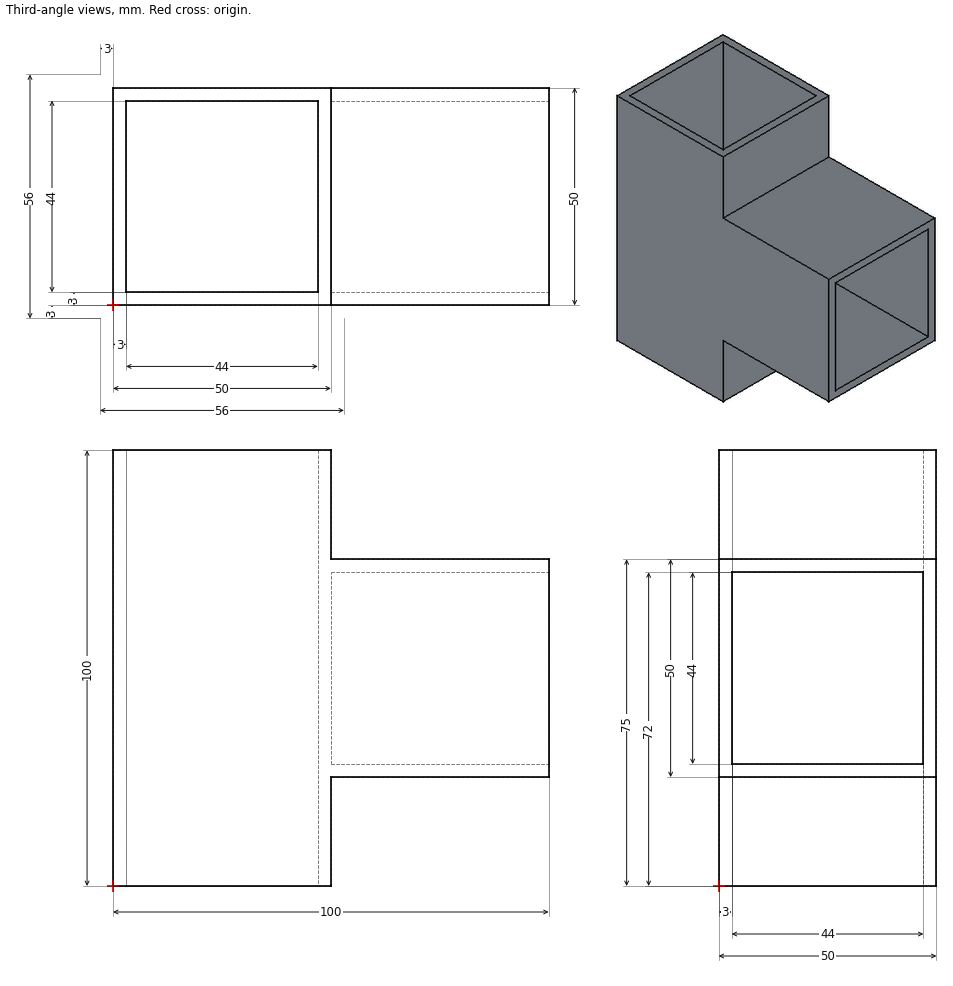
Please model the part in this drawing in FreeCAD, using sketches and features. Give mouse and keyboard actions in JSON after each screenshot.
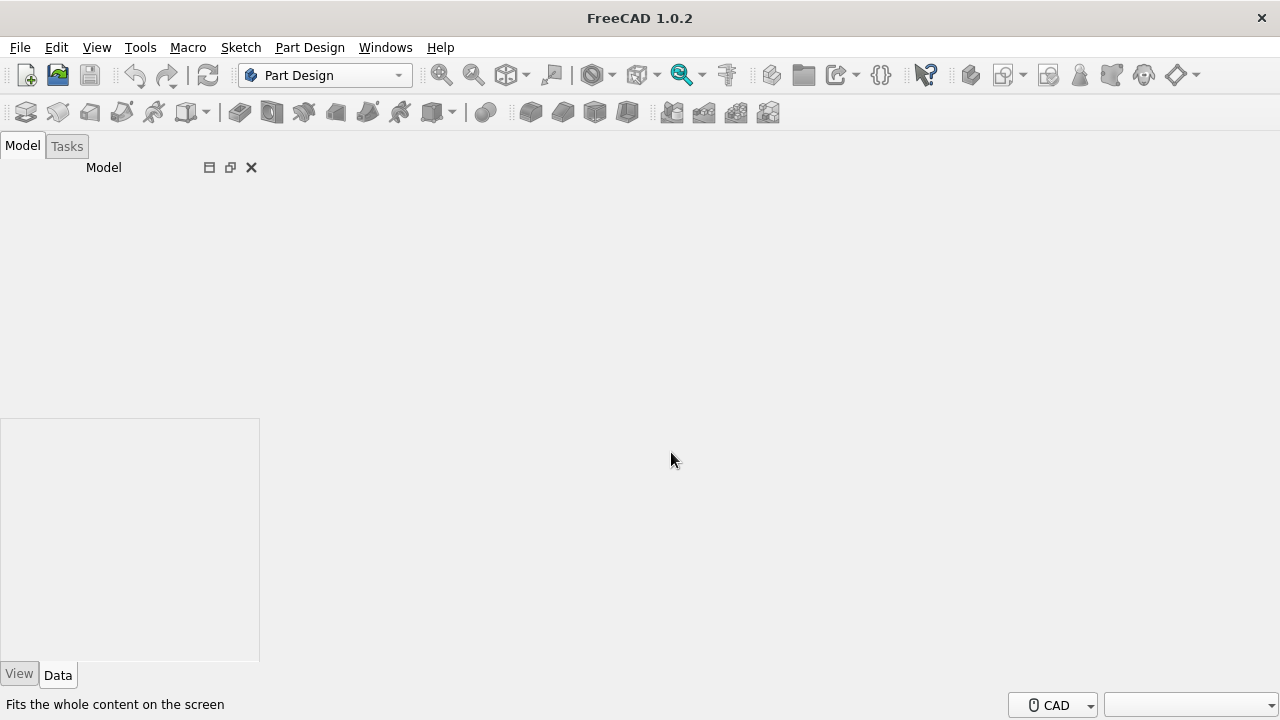
{"action": "left_click", "coordinate": [26, 76]}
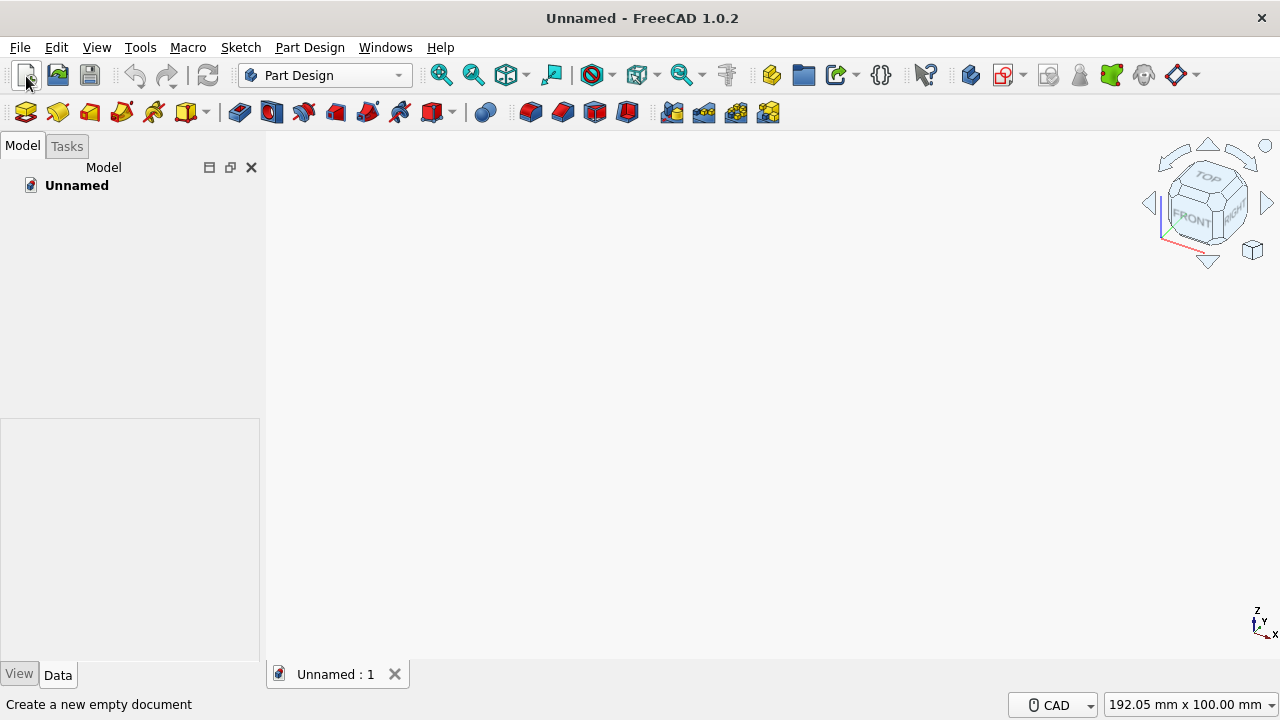
{"action": "left_click", "coordinate": [1004, 76]}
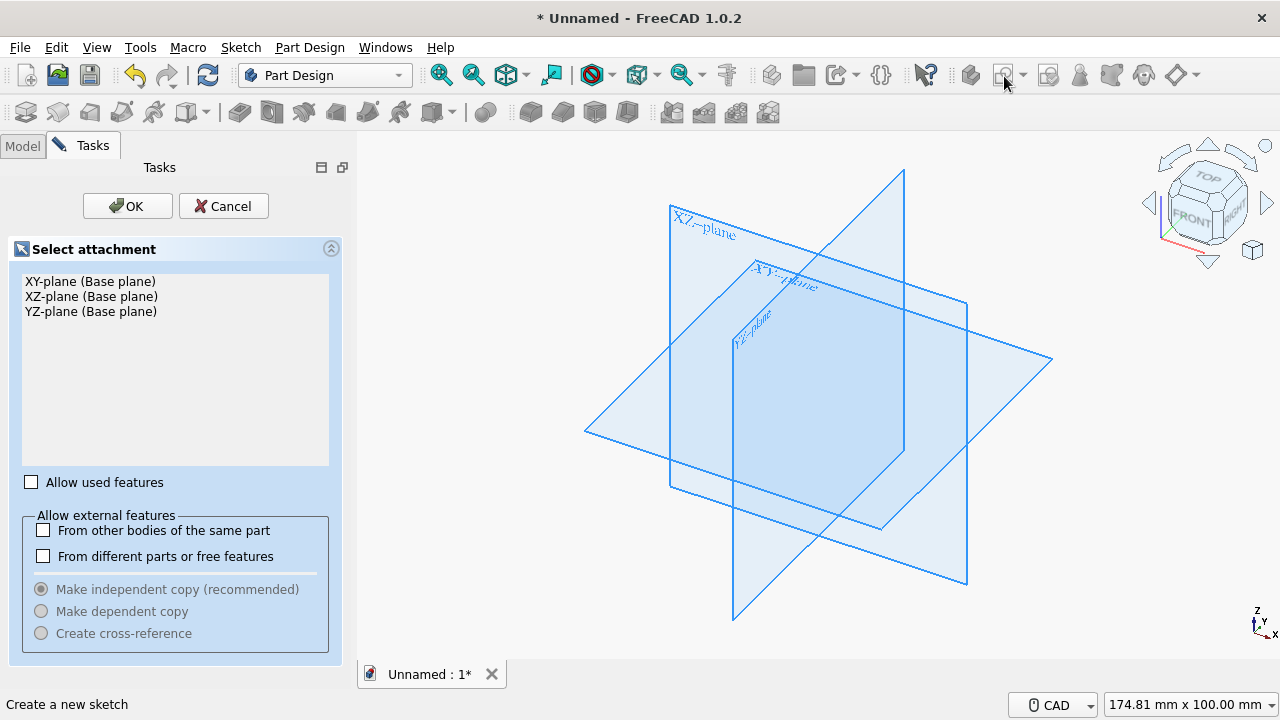
{"action": "left_click", "coordinate": [82, 282]}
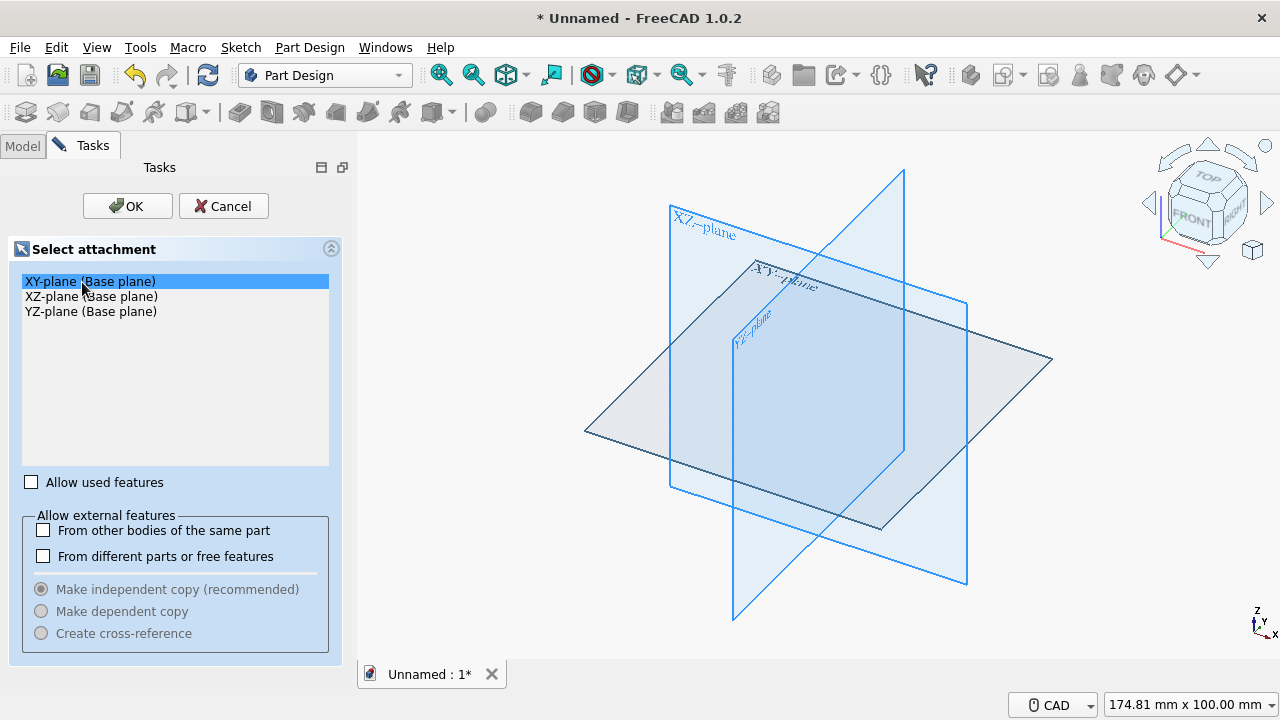
{"action": "left_click", "coordinate": [128, 206]}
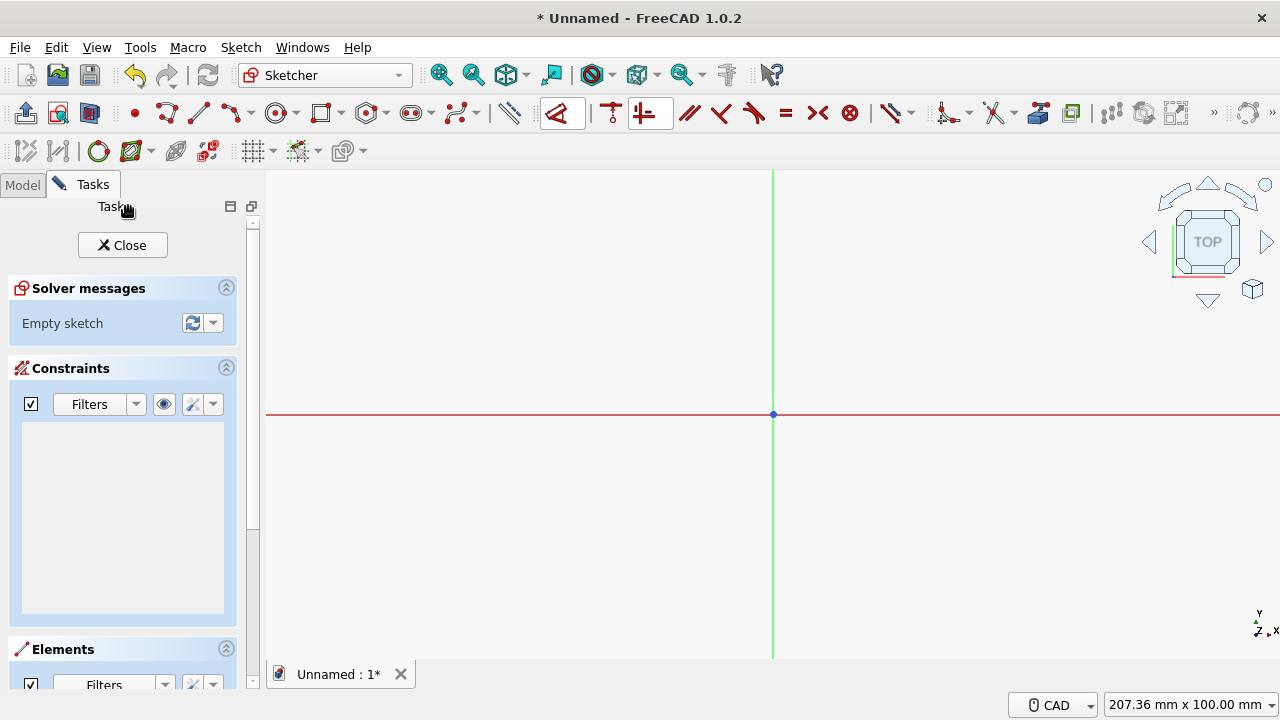
{"action": "scroll", "coordinate": [294, 631], "scroll_direction": "down", "scroll_amount": 1}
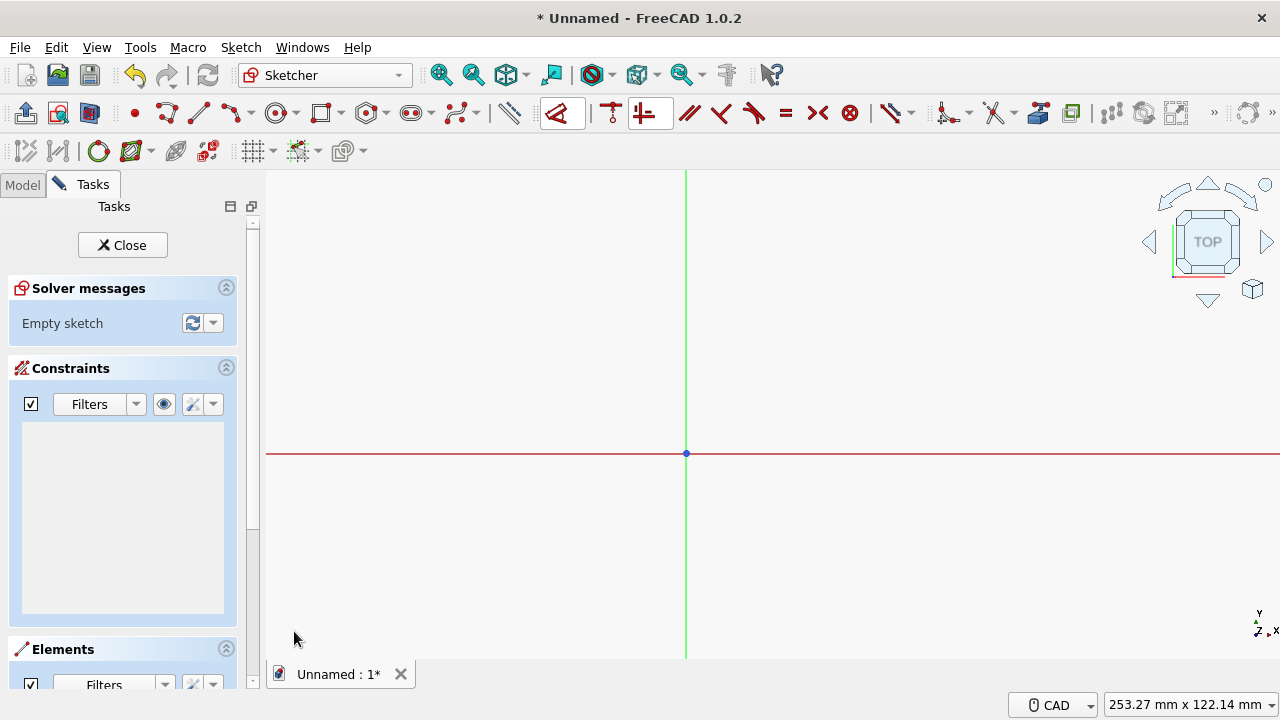
{"action": "scroll", "coordinate": [953, 230], "scroll_direction": "up", "scroll_amount": 2}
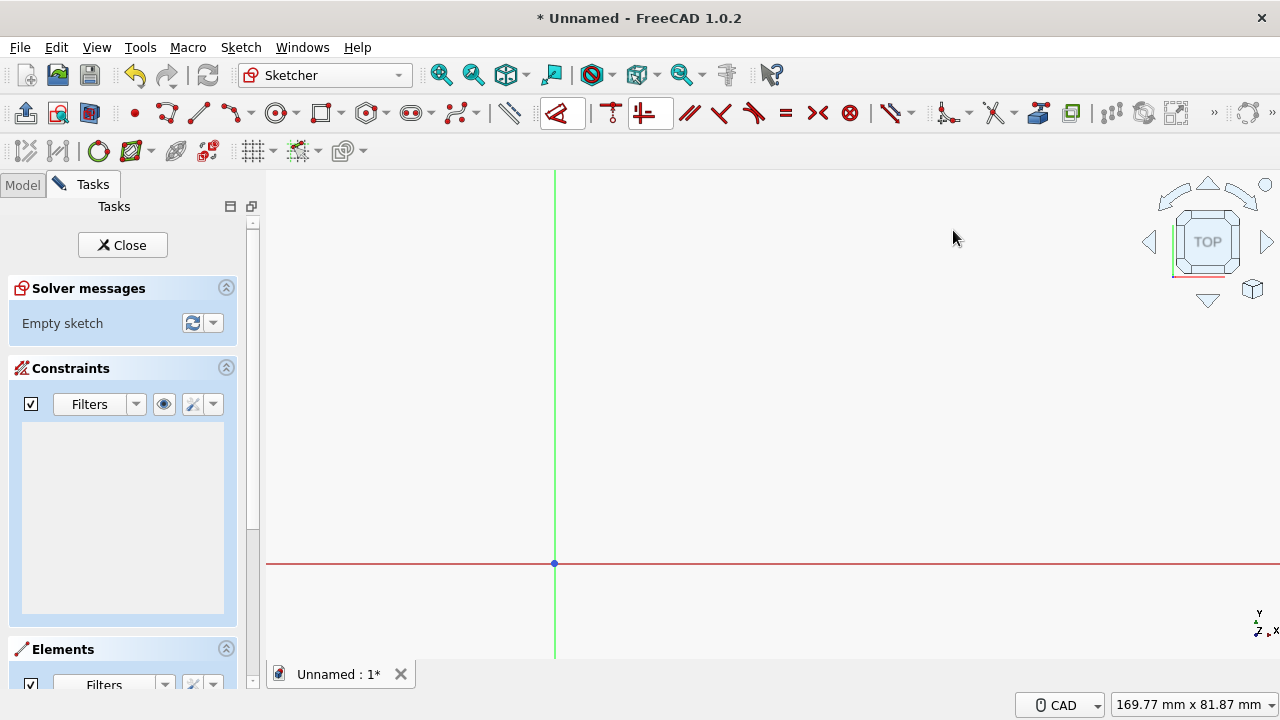
{"action": "left_click", "coordinate": [322, 114]}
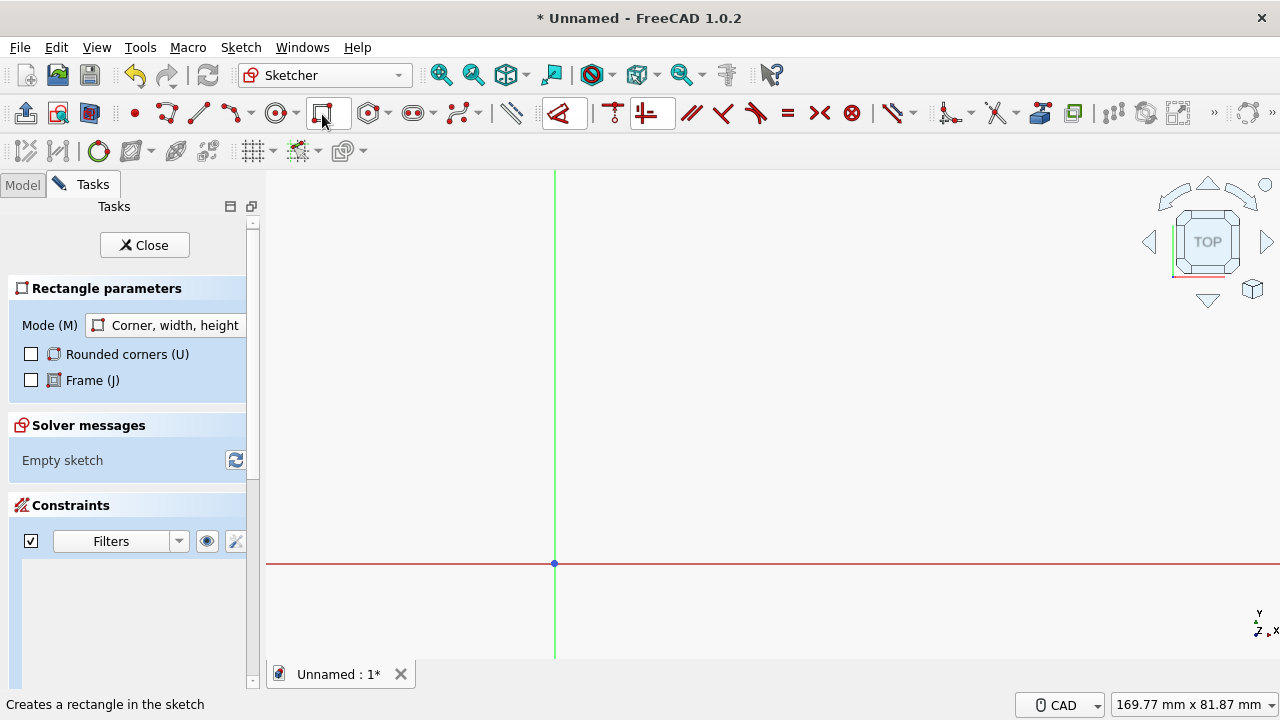
{"action": "left_click", "coordinate": [555, 564]}
{"action": "left_click", "coordinate": [853, 265]}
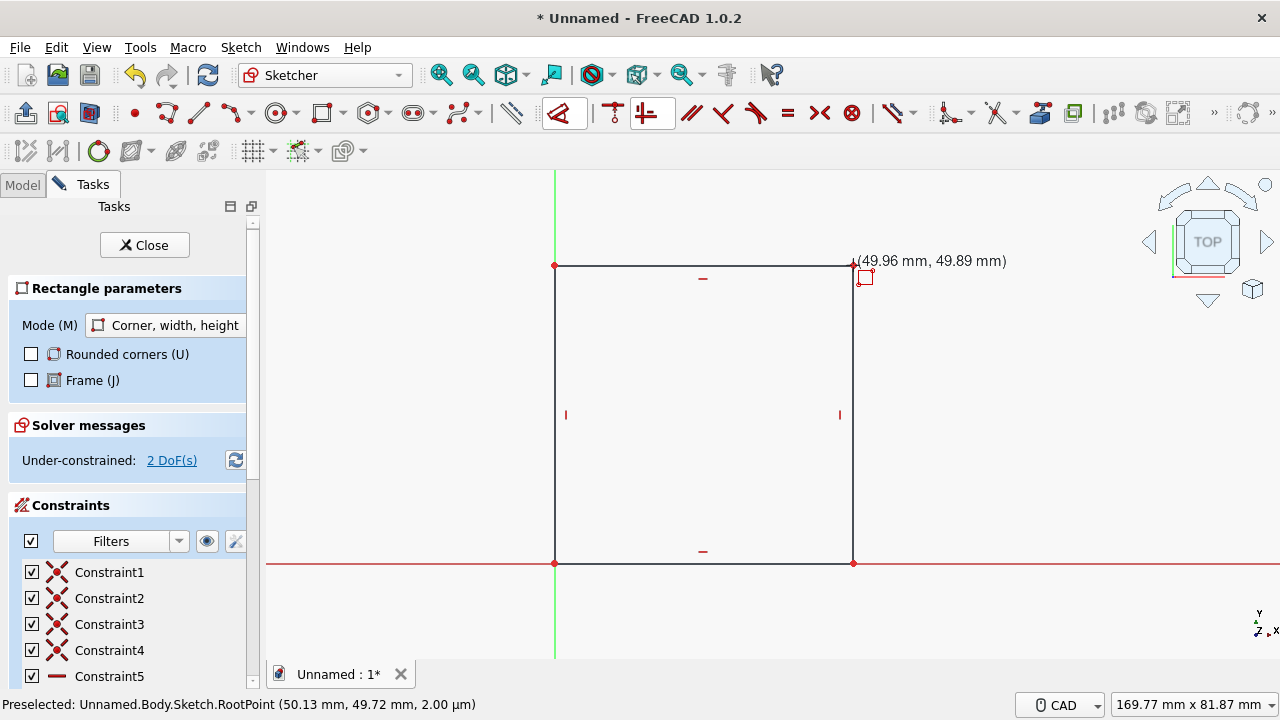
{"action": "left_click", "coordinate": [573, 283]}
{"action": "left_click", "coordinate": [835, 546]}
{"action": "key", "text": "Escape"}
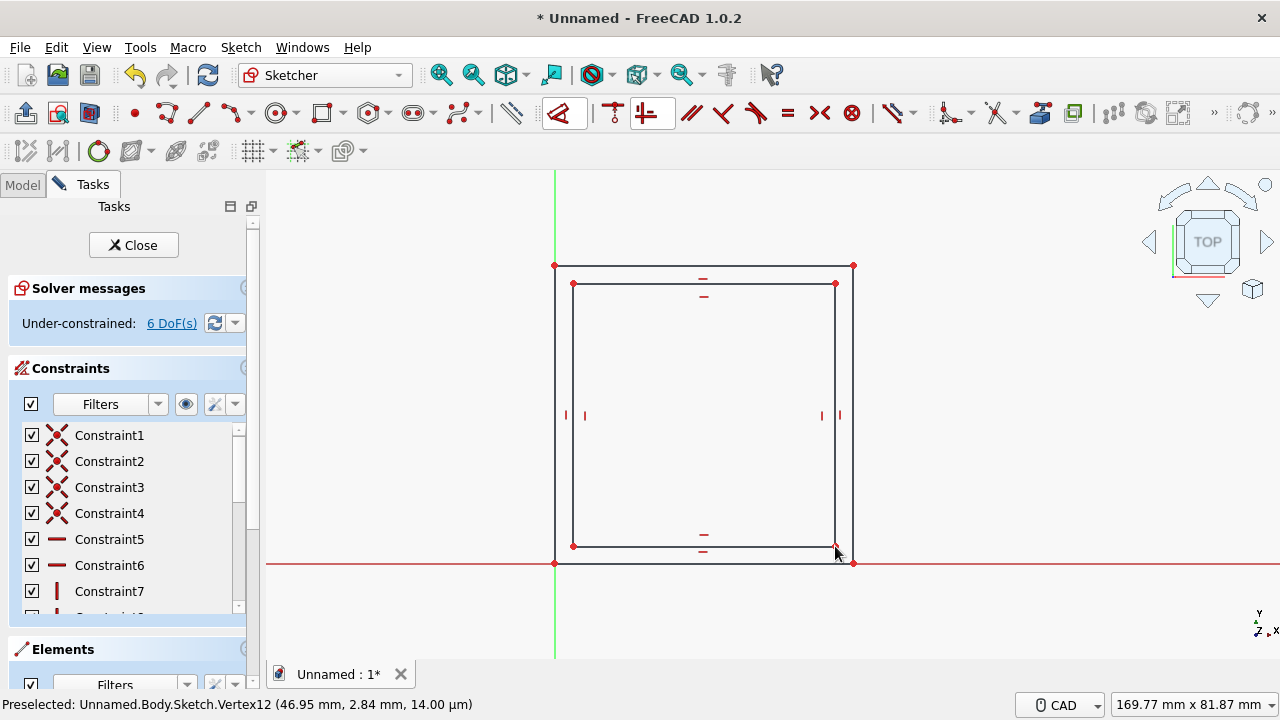
{"action": "left_click", "coordinate": [644, 564]}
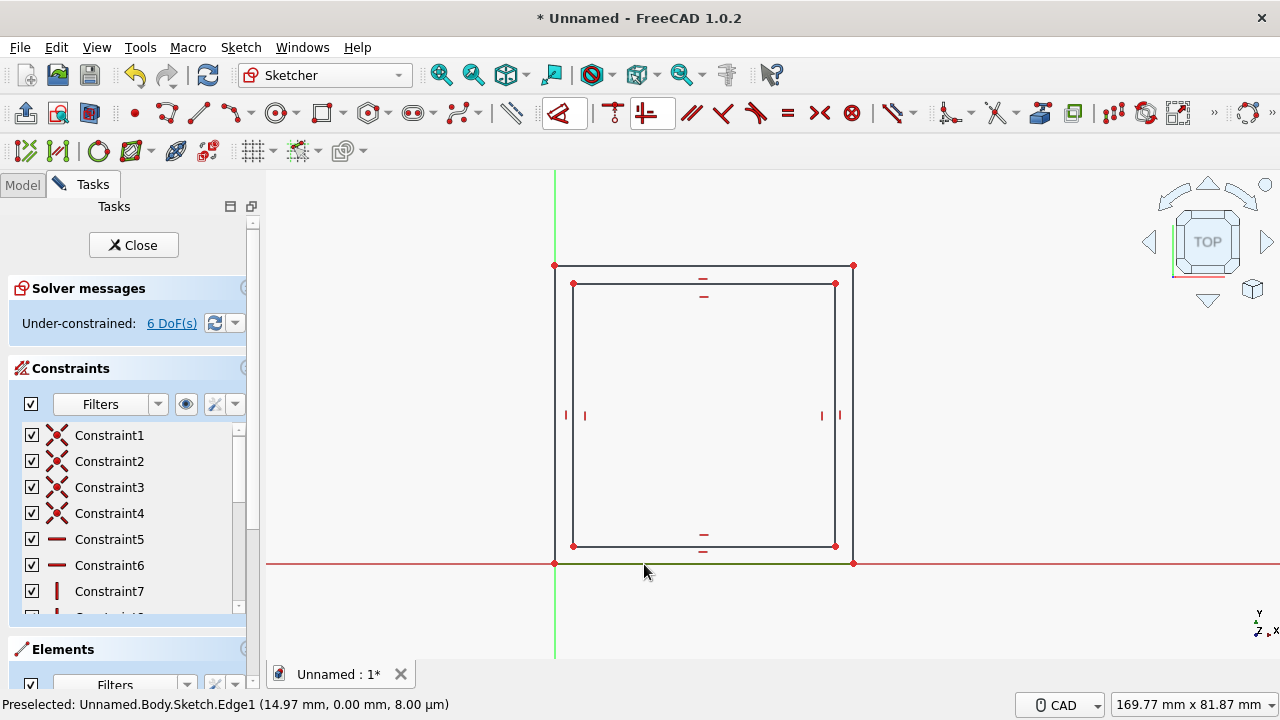
{"action": "key", "text": "l"}